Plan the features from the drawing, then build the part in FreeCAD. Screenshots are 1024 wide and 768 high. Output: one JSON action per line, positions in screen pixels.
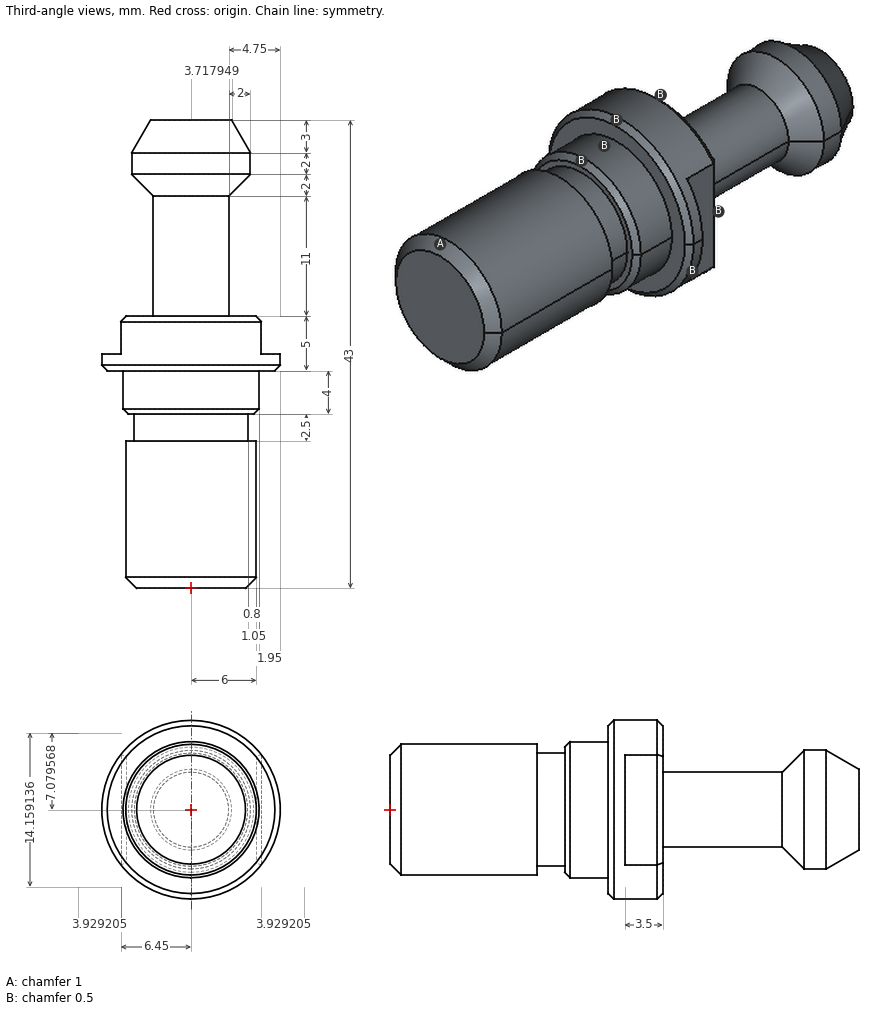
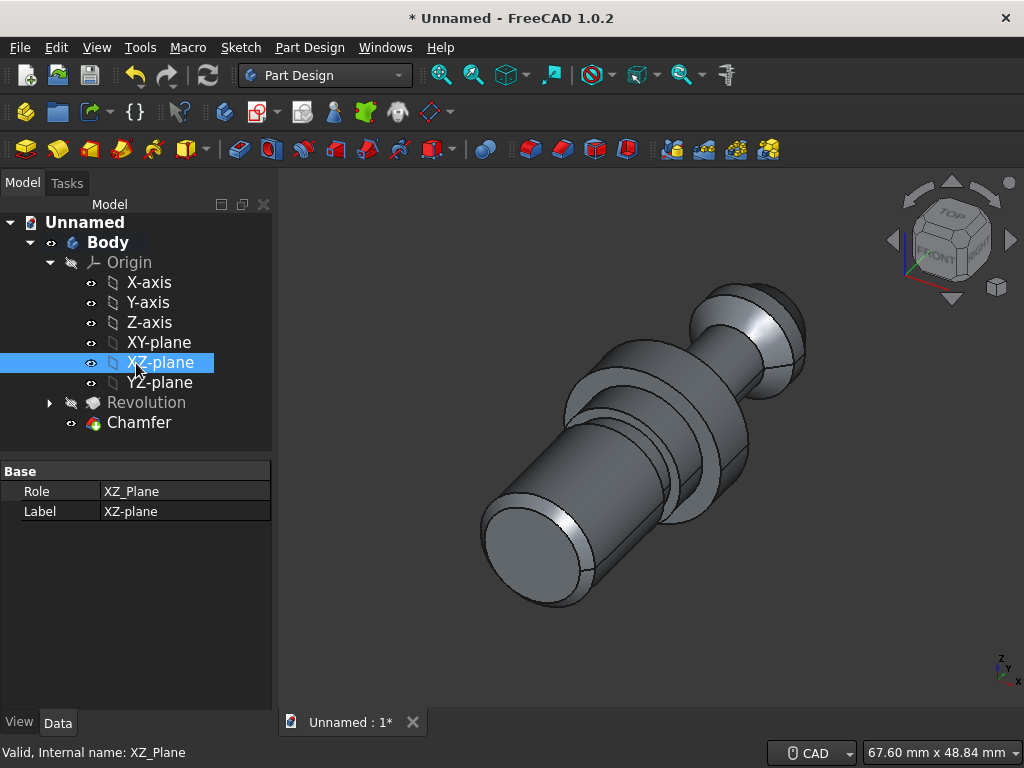
{"action": "left_click", "coordinate": [430, 112]}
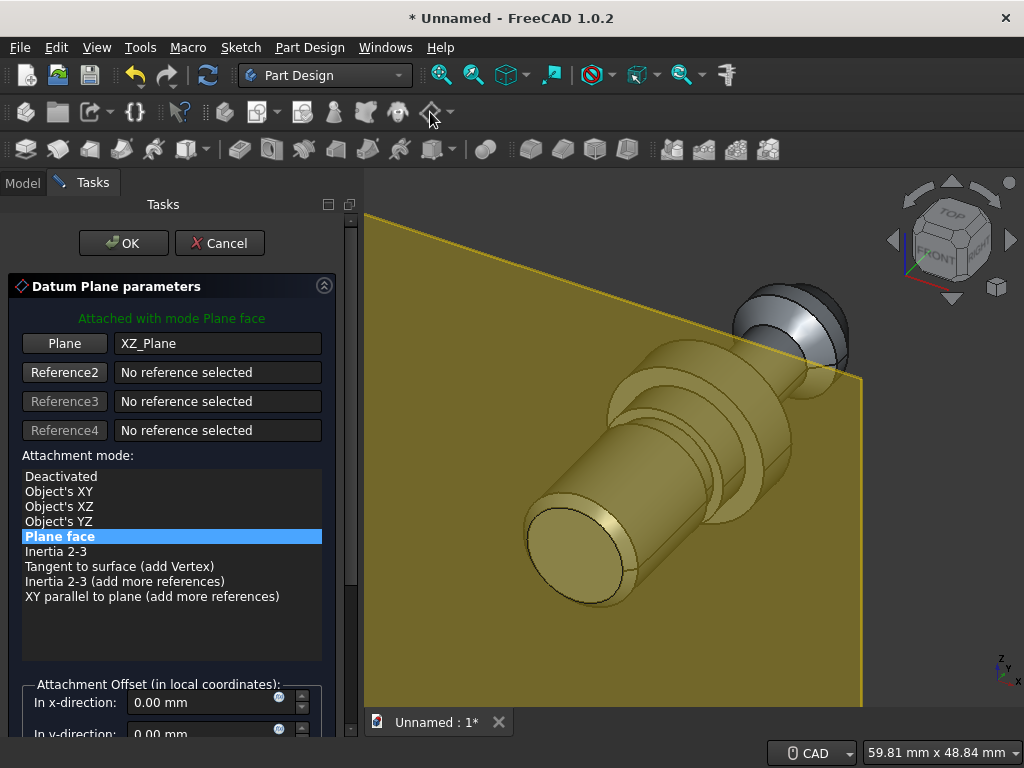
{"action": "scroll", "coordinate": [351, 475], "scroll_direction": "down", "scroll_amount": 2}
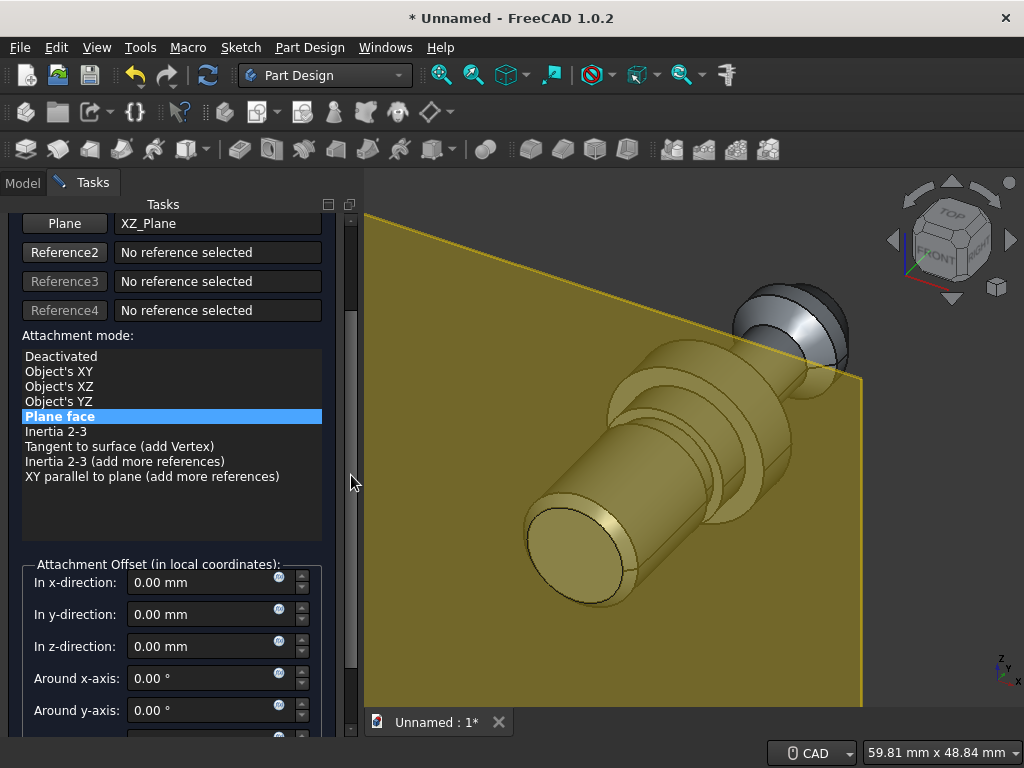
{"action": "triple_click", "coordinate": [210, 646]}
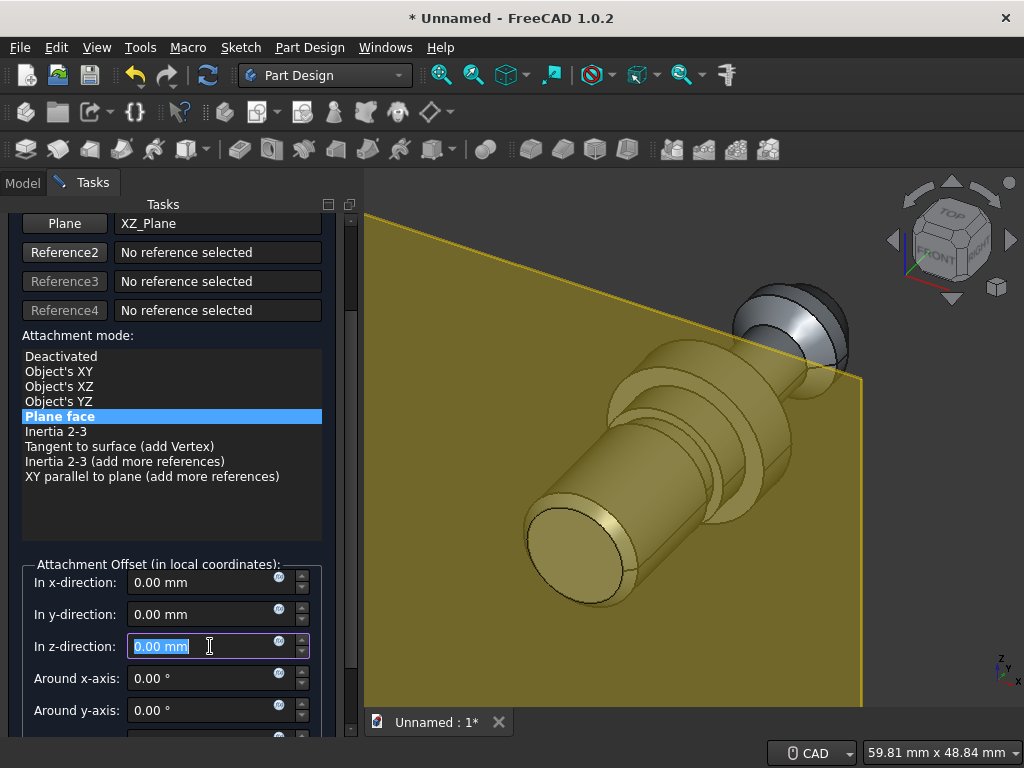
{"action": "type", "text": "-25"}
{"action": "key", "text": "Tab"}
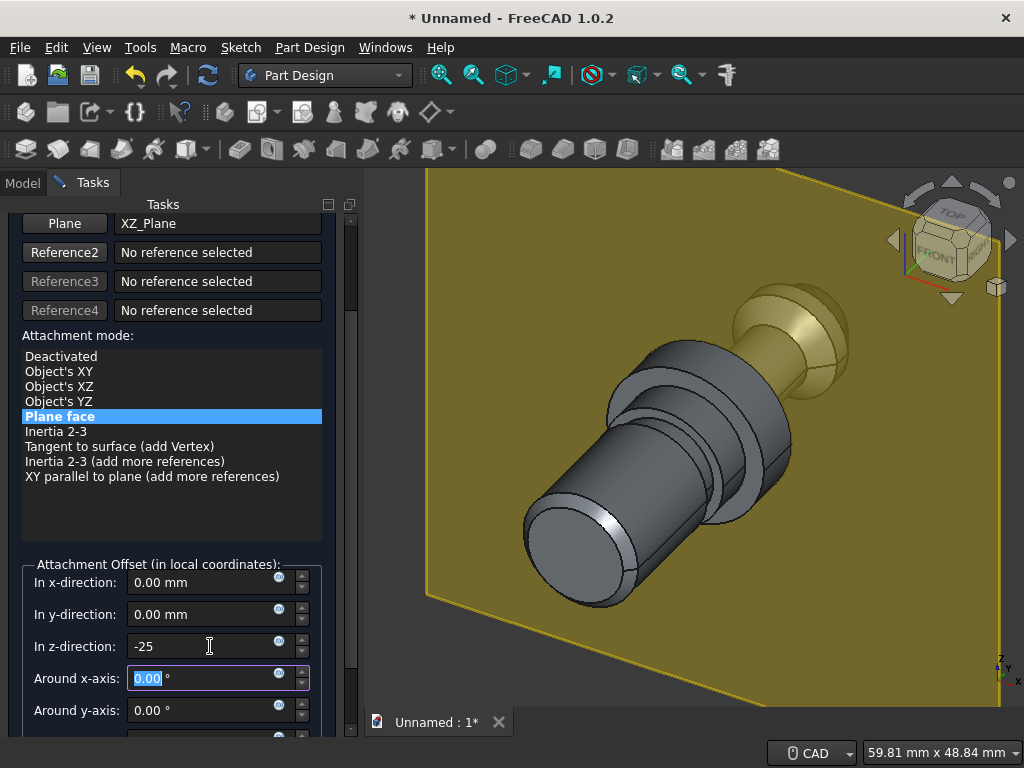
{"action": "scroll", "coordinate": [351, 475], "scroll_direction": "up", "scroll_amount": 3}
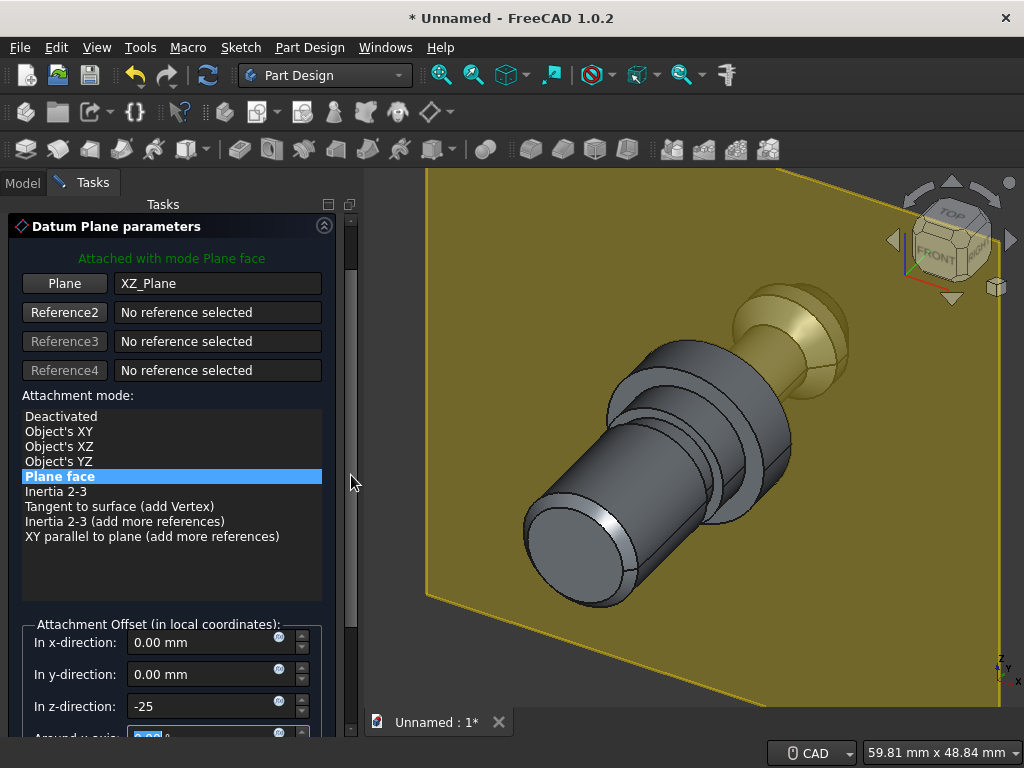
{"action": "left_click", "coordinate": [124, 243]}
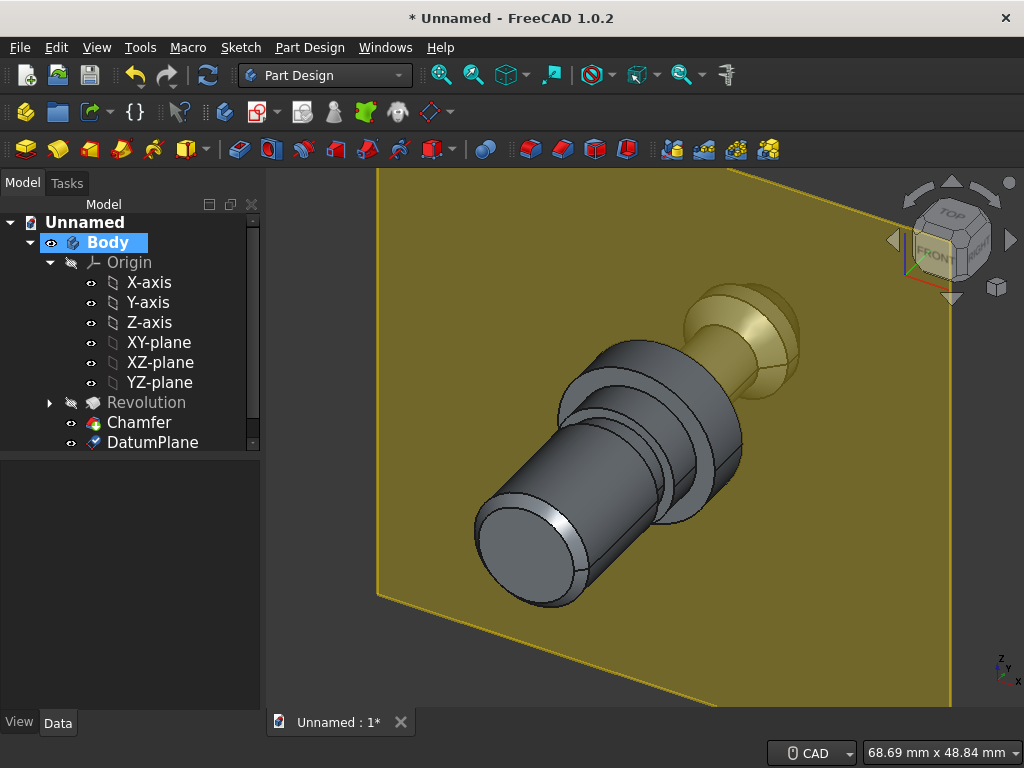
{"action": "left_click", "coordinate": [116, 443]}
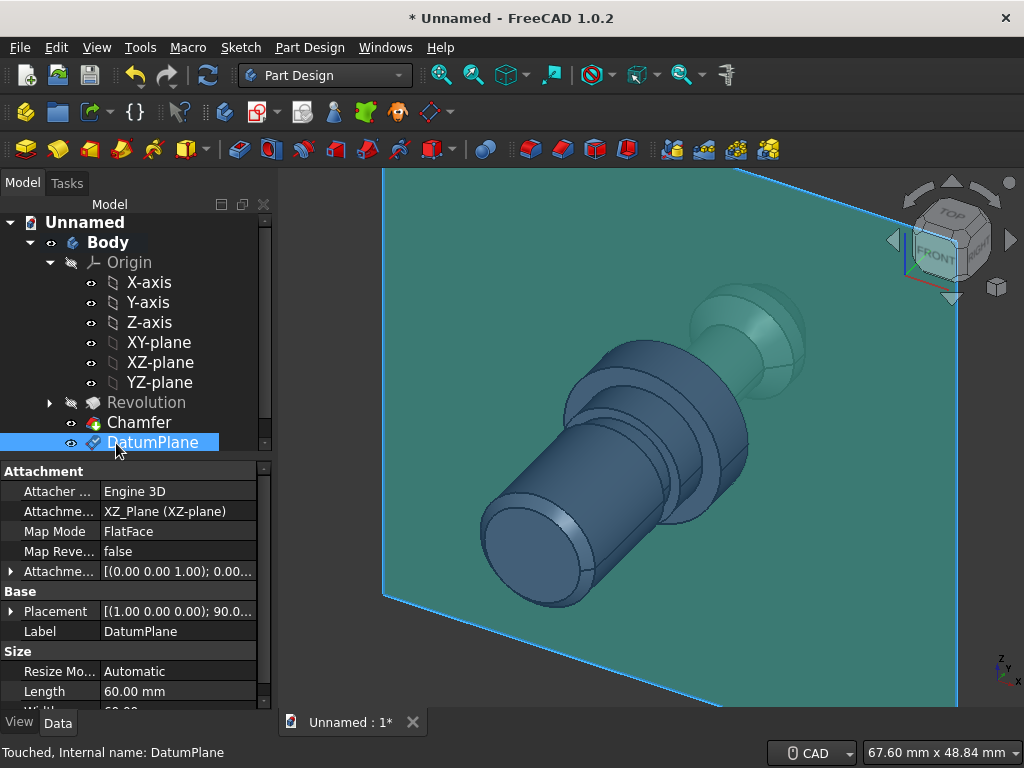
{"action": "left_click", "coordinate": [258, 112]}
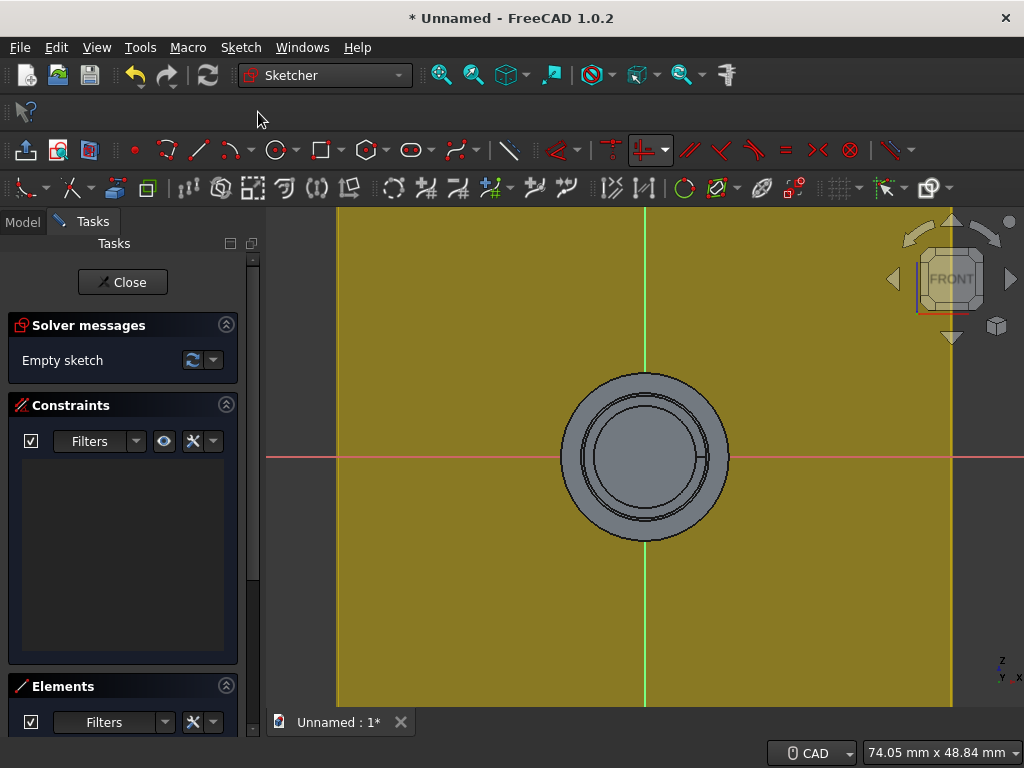
{"action": "left_click", "coordinate": [90, 150]}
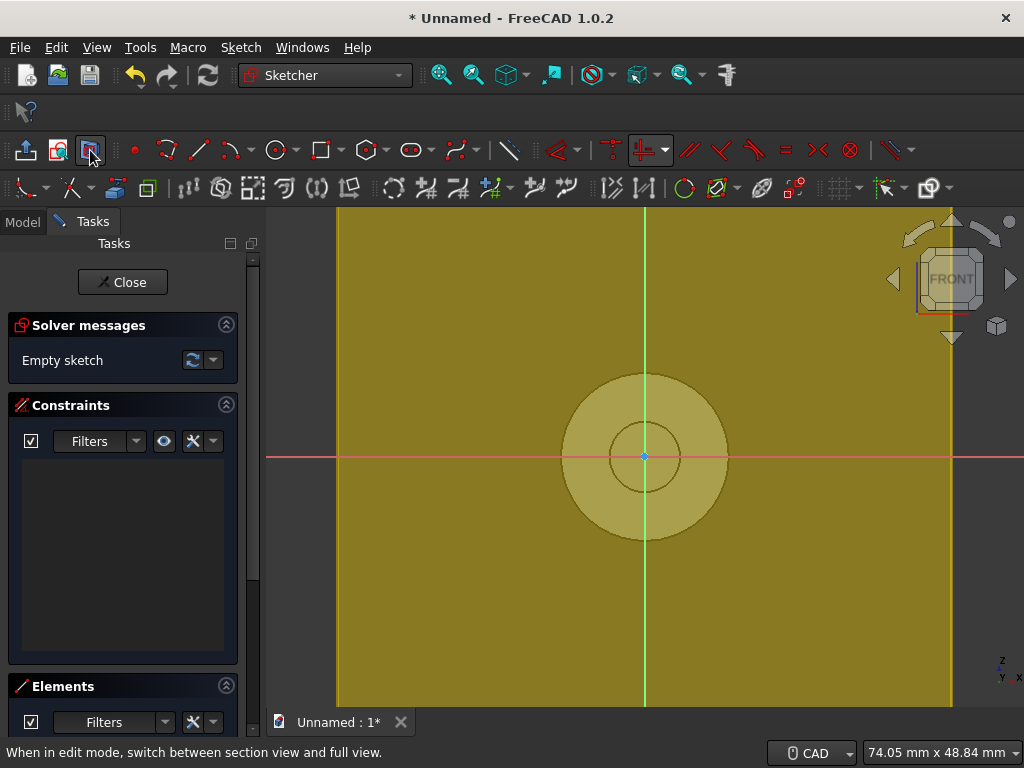
{"action": "scroll", "coordinate": [728, 457], "scroll_direction": "up", "scroll_amount": 3}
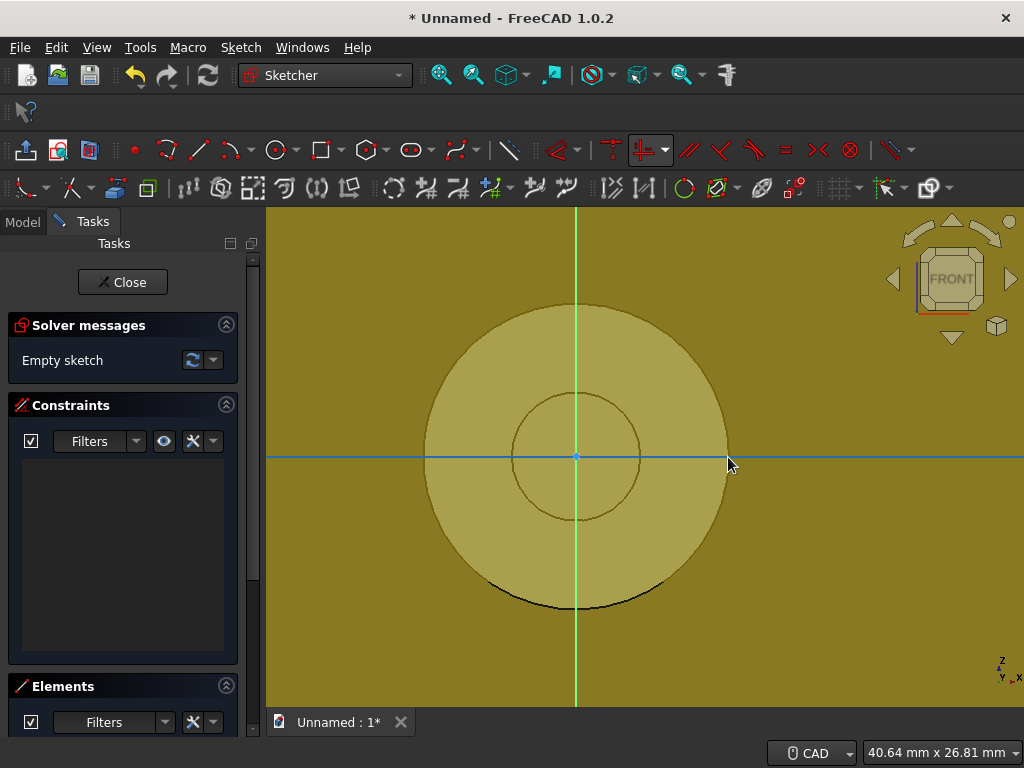
{"action": "left_click", "coordinate": [322, 150]}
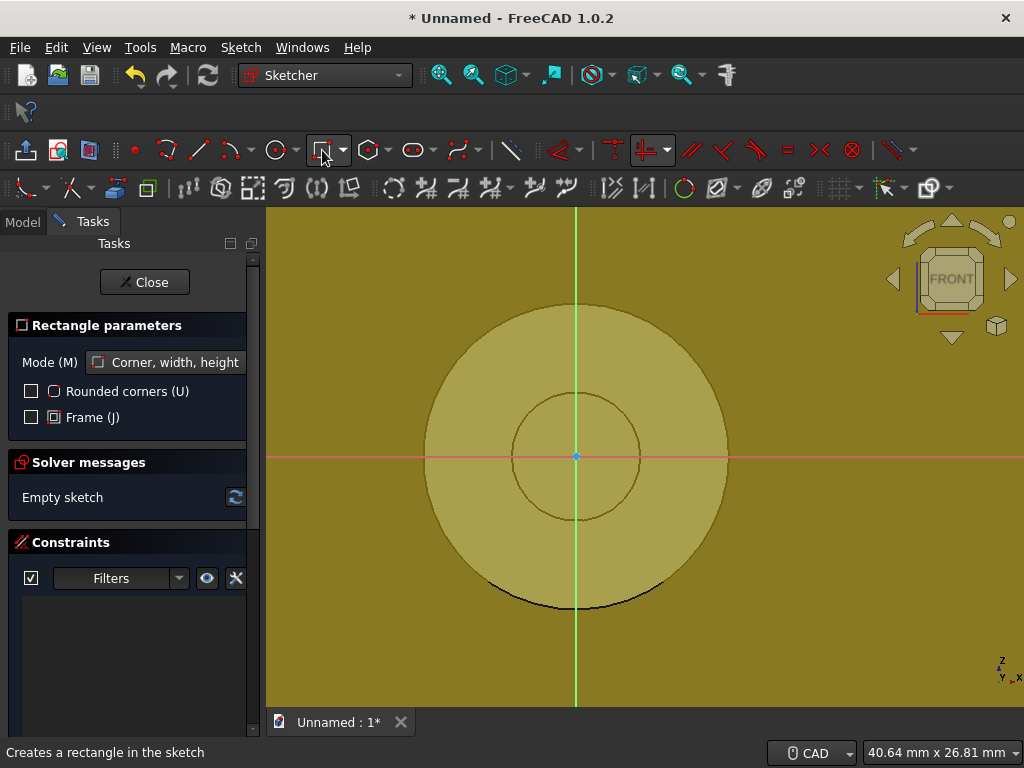
{"action": "left_click", "coordinate": [382, 325]}
{"action": "mouse_move", "coordinate": [456, 589]}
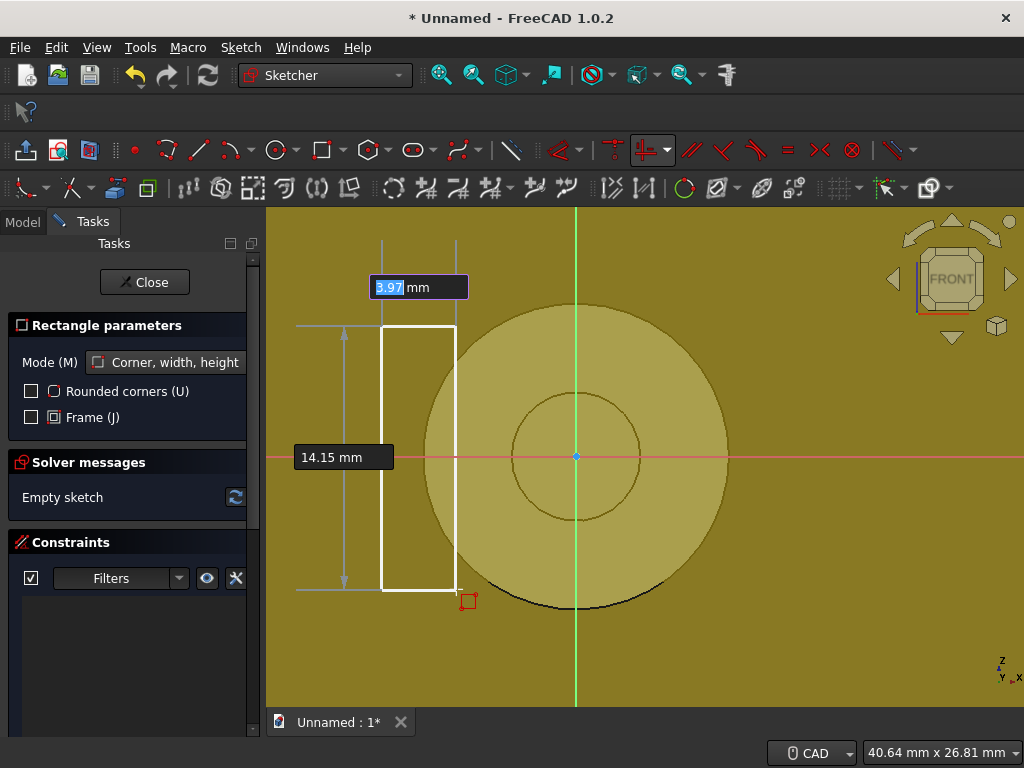
{"action": "type", "text": "3.929205"}
{"action": "key", "text": "Tab"}
{"action": "type", "text": "14.159136"}
{"action": "key", "text": "Return"}